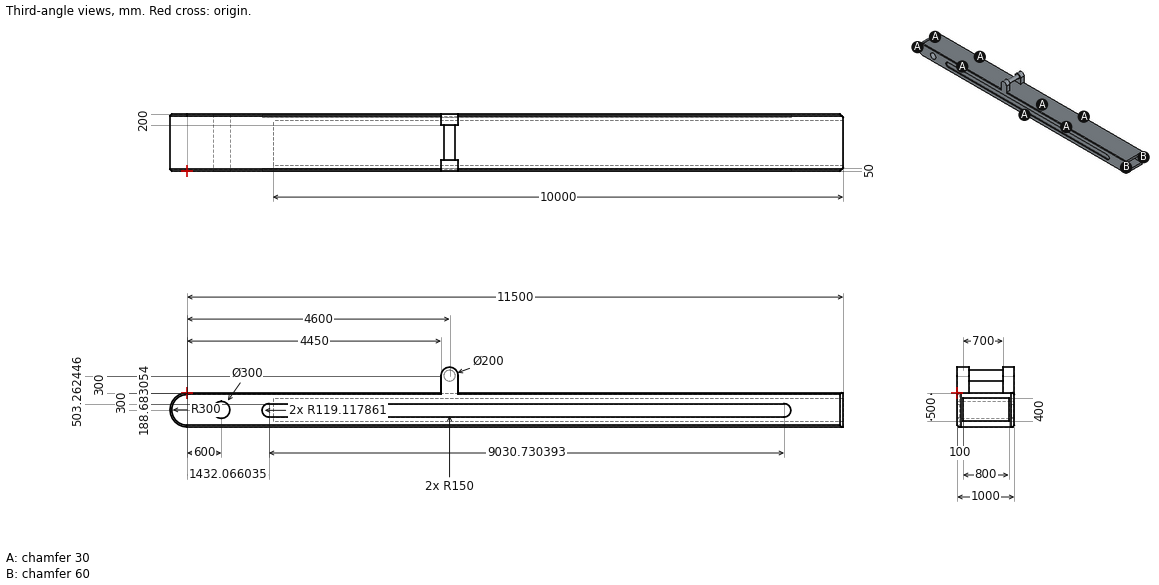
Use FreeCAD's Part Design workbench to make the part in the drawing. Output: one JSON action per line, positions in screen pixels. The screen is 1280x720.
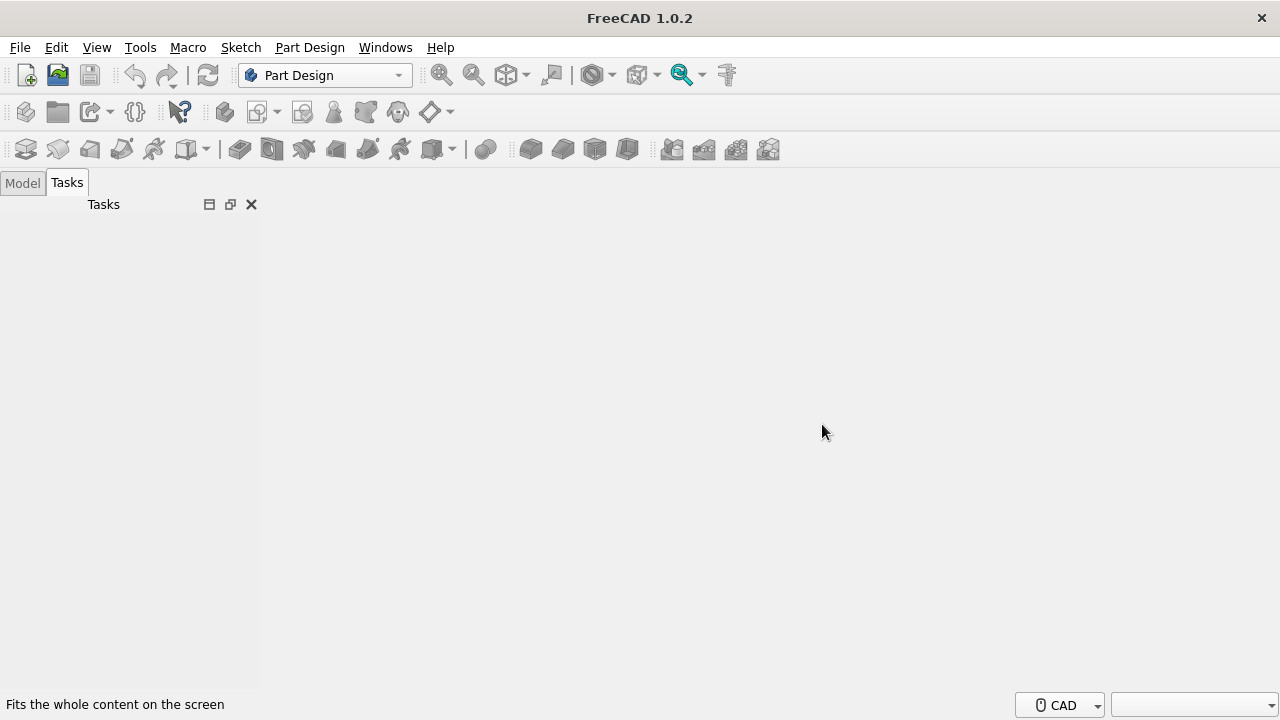
{"action": "left_click", "coordinate": [26, 76]}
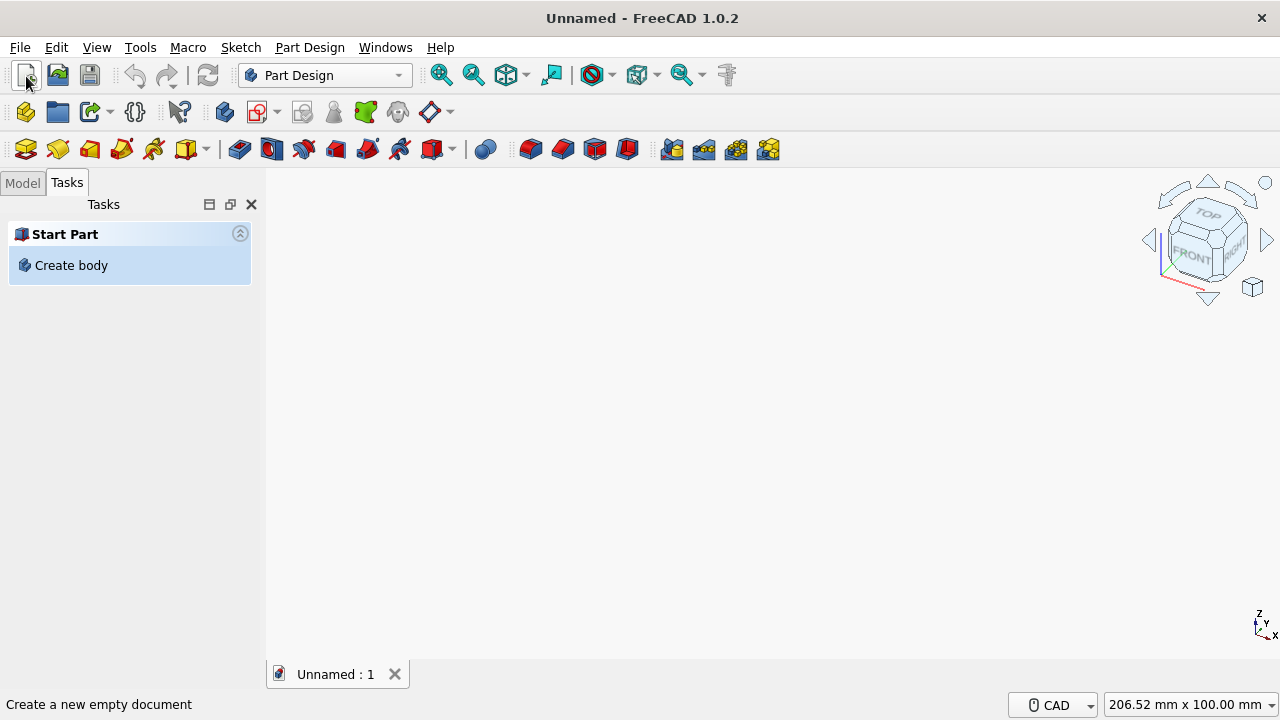
{"action": "left_click", "coordinate": [258, 112]}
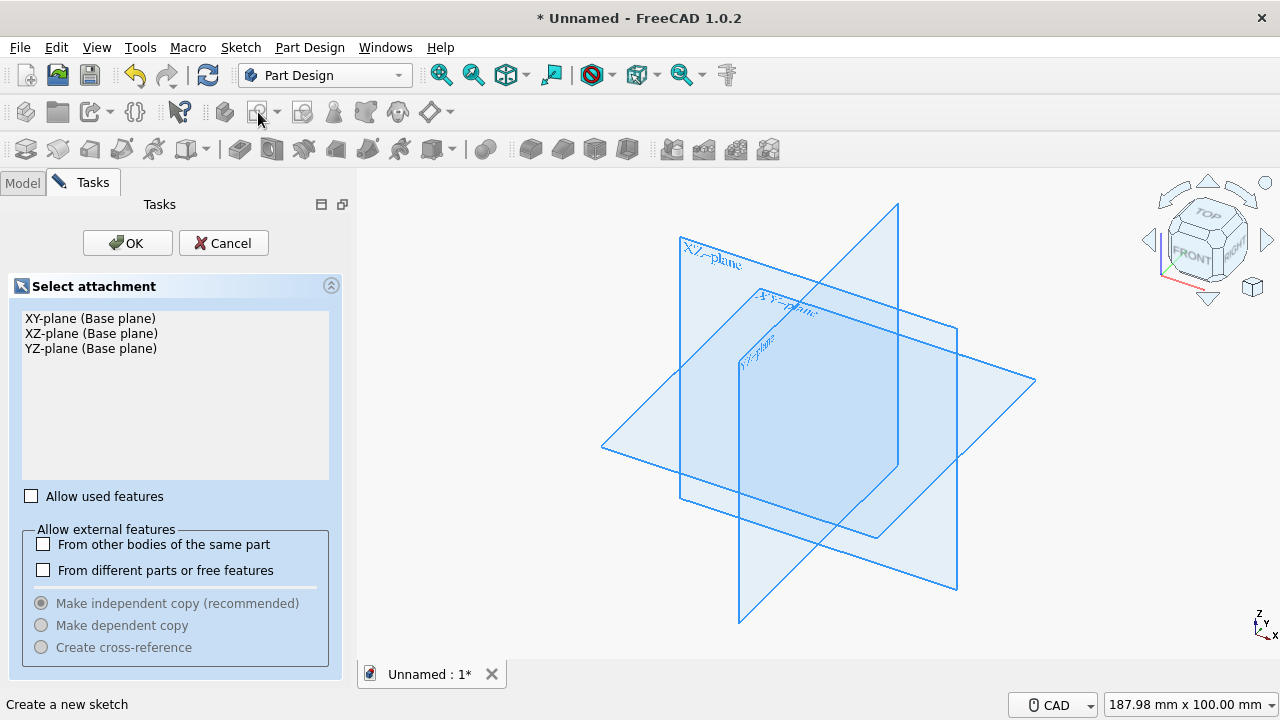
{"action": "left_click", "coordinate": [82, 334]}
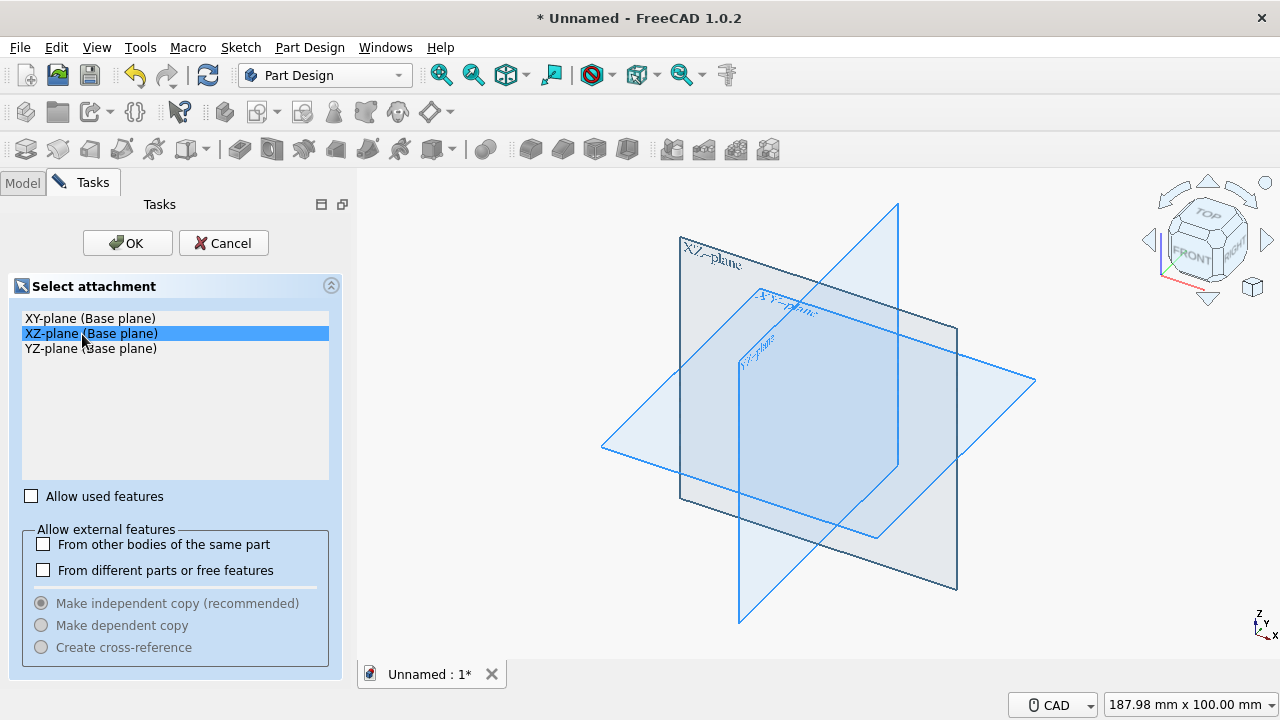
{"action": "left_click", "coordinate": [128, 243]}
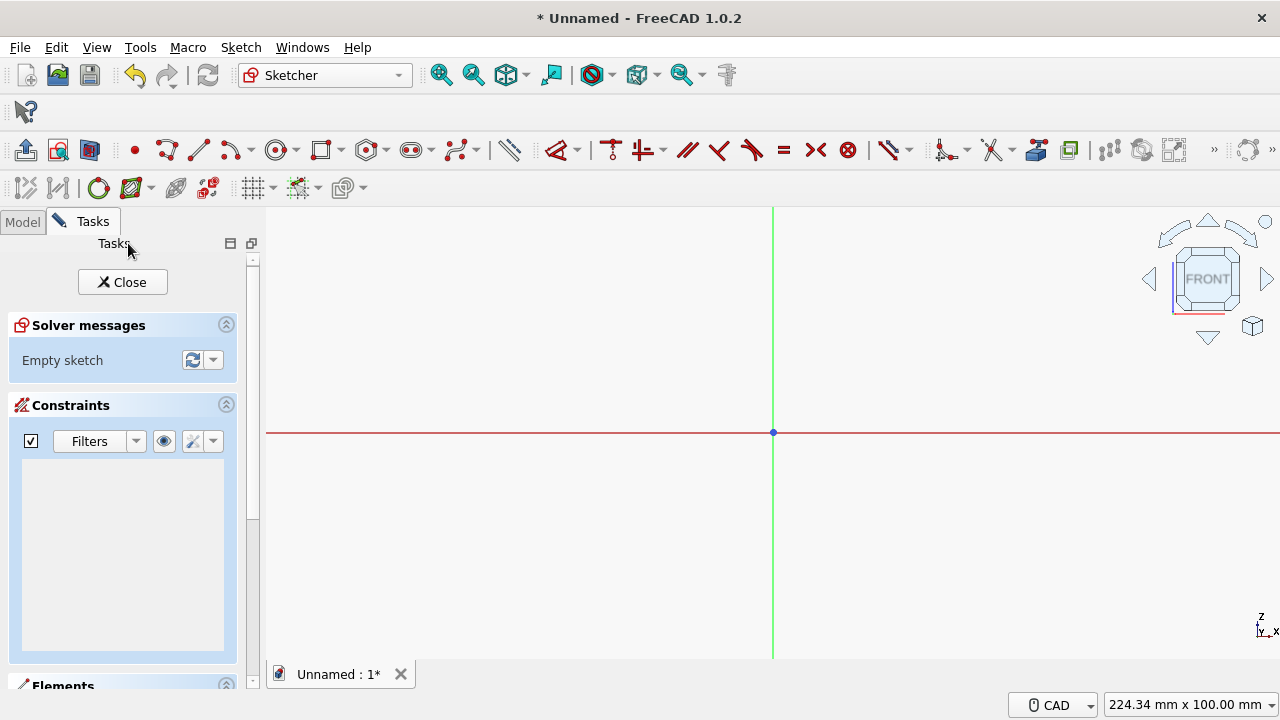
{"action": "scroll", "coordinate": [704, 433], "scroll_direction": "down", "scroll_amount": 15}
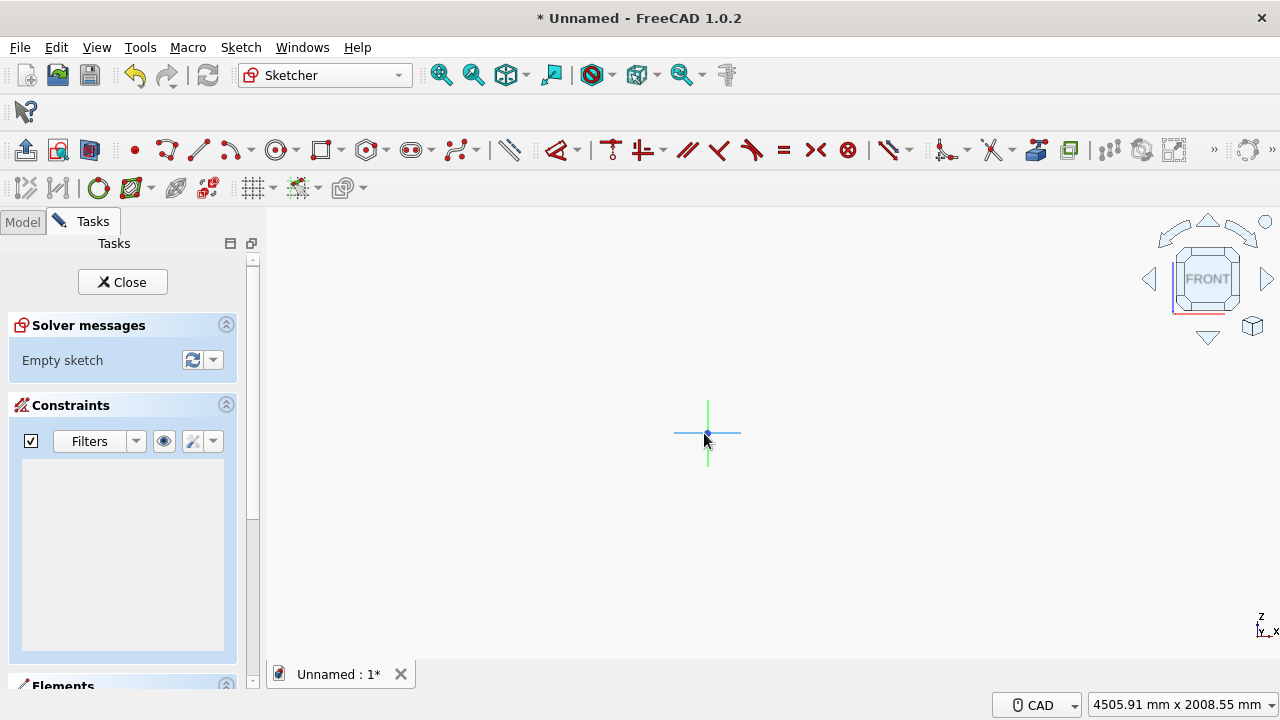
{"action": "scroll", "coordinate": [385, 416], "scroll_direction": "down", "scroll_amount": 8}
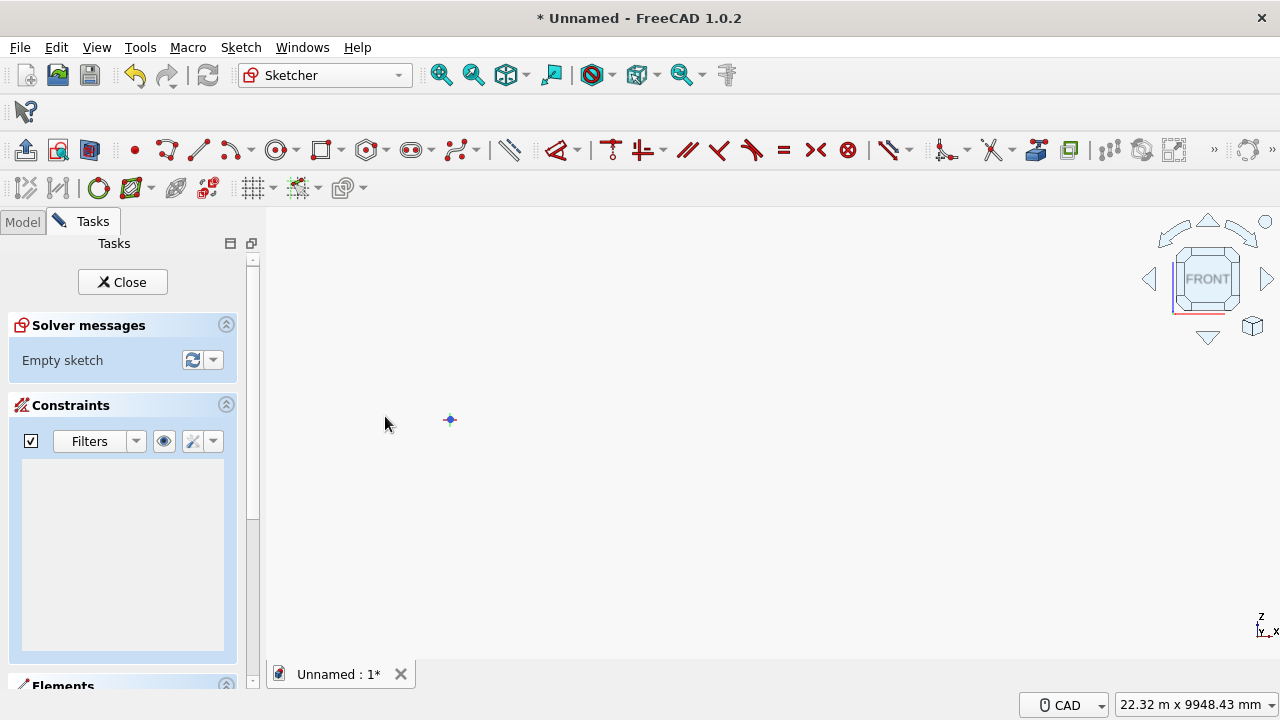
{"action": "left_click", "coordinate": [168, 150]}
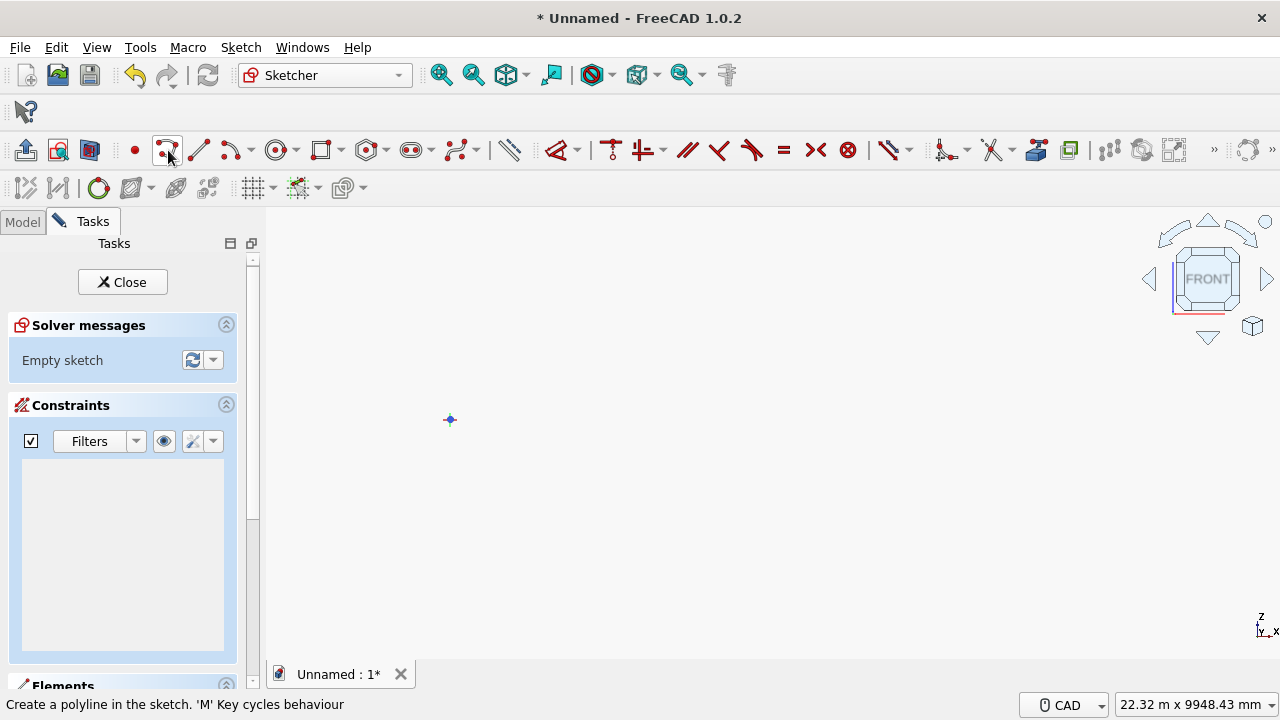
{"action": "left_click", "coordinate": [450, 420]}
{"action": "left_click", "coordinate": [973, 429]}
{"action": "left_click", "coordinate": [973, 447]}
{"action": "left_click", "coordinate": [450, 447]}
{"action": "right_click", "coordinate": [450, 447]}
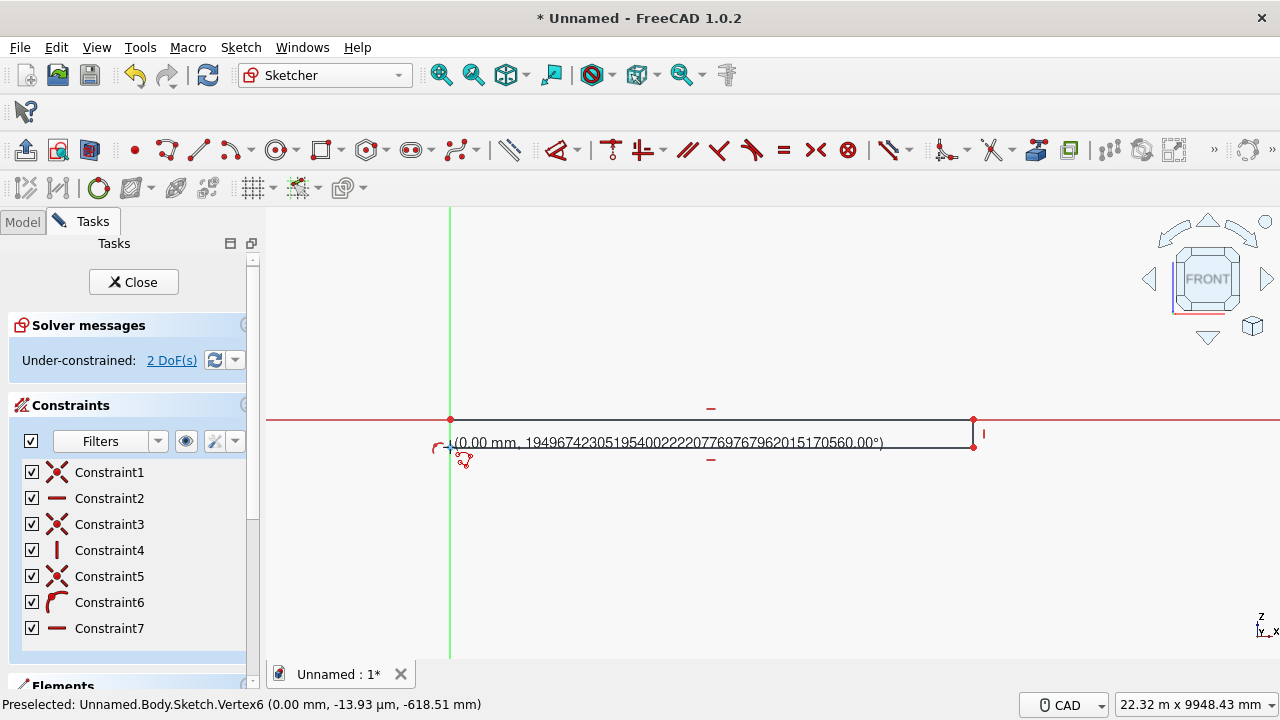
{"action": "left_click", "coordinate": [254, 150]}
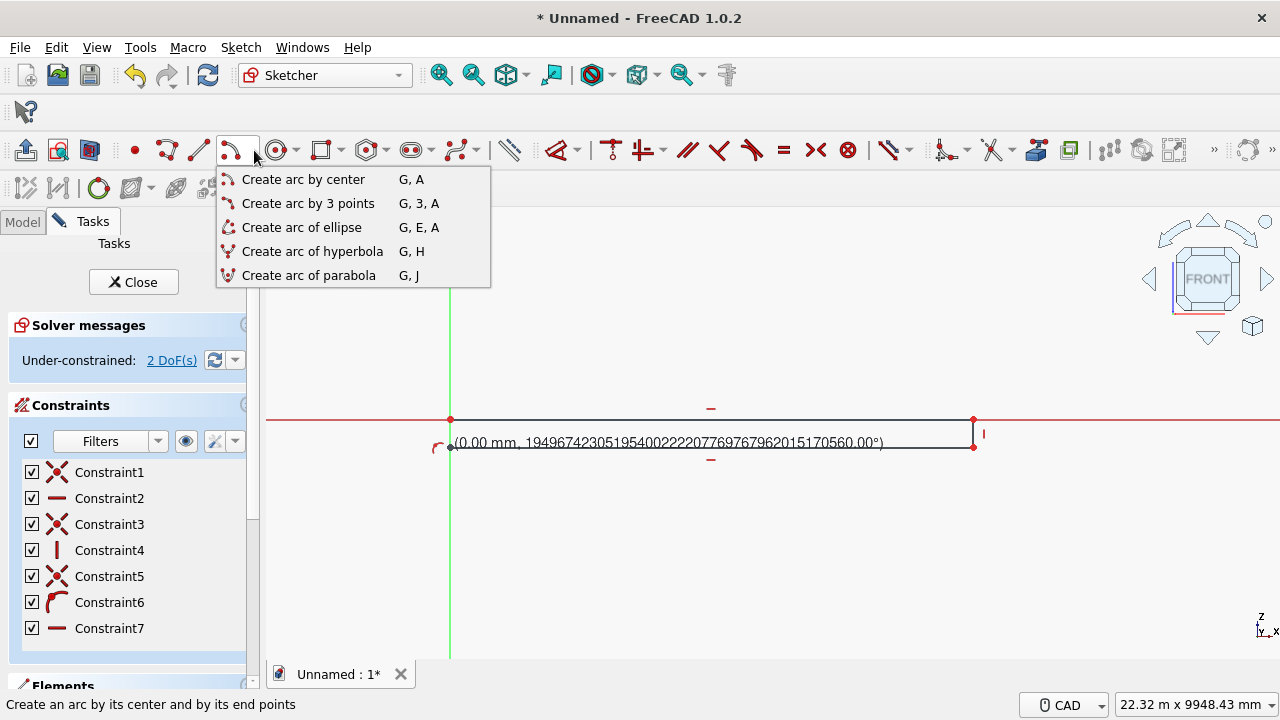
{"action": "left_click", "coordinate": [354, 203]}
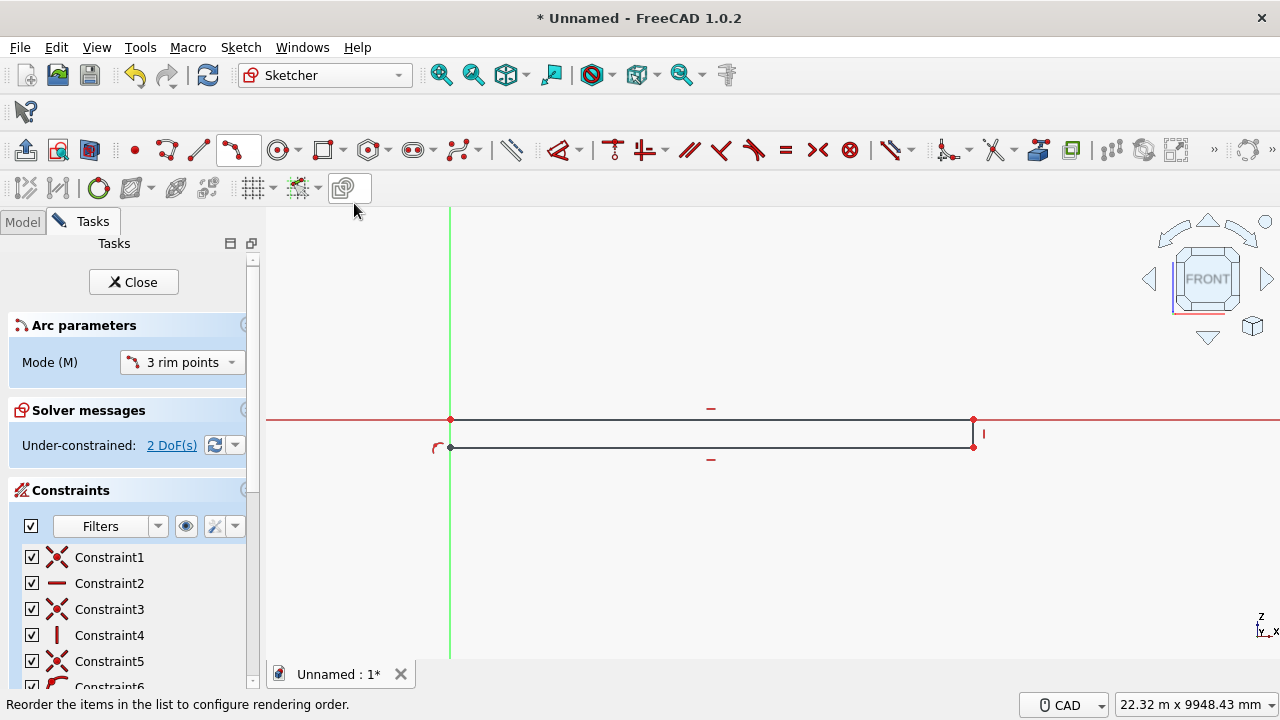
{"action": "left_click", "coordinate": [450, 448]}
{"action": "left_click", "coordinate": [450, 420]}
{"action": "left_click", "coordinate": [437, 434]}